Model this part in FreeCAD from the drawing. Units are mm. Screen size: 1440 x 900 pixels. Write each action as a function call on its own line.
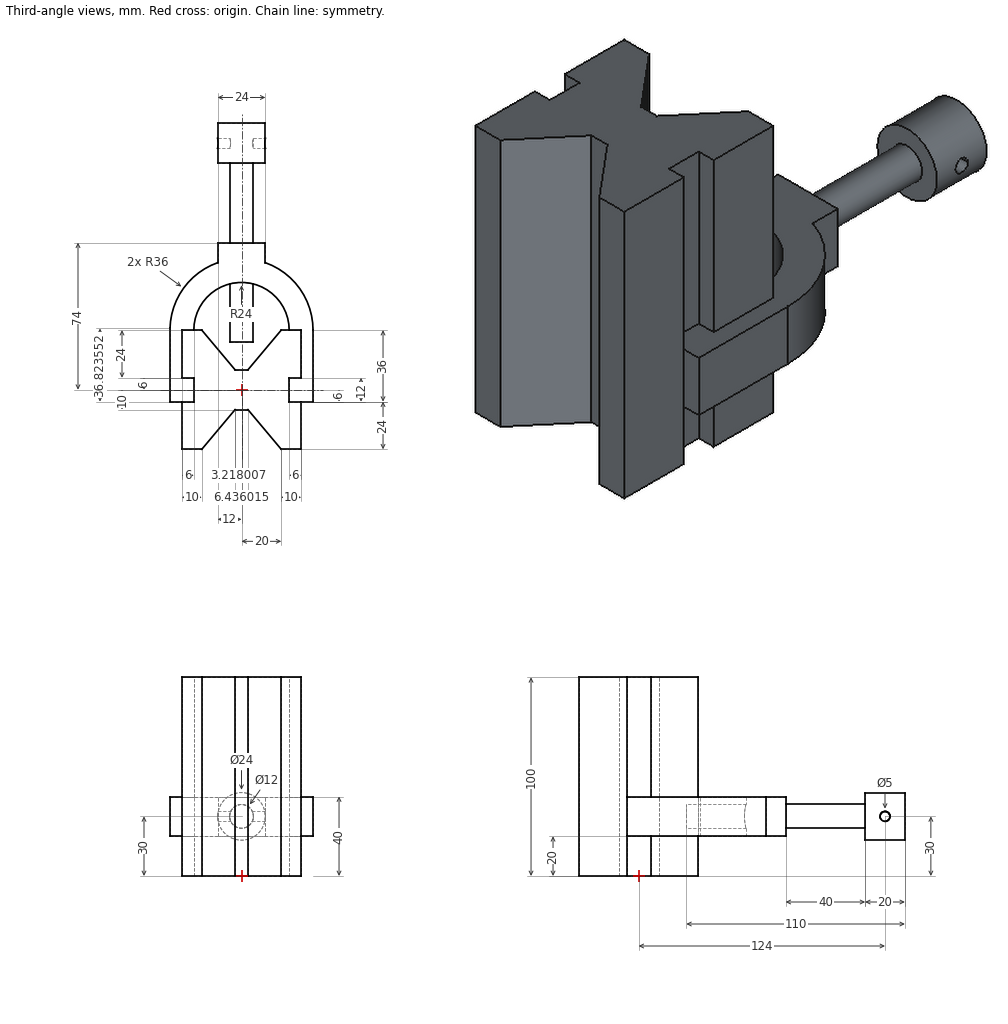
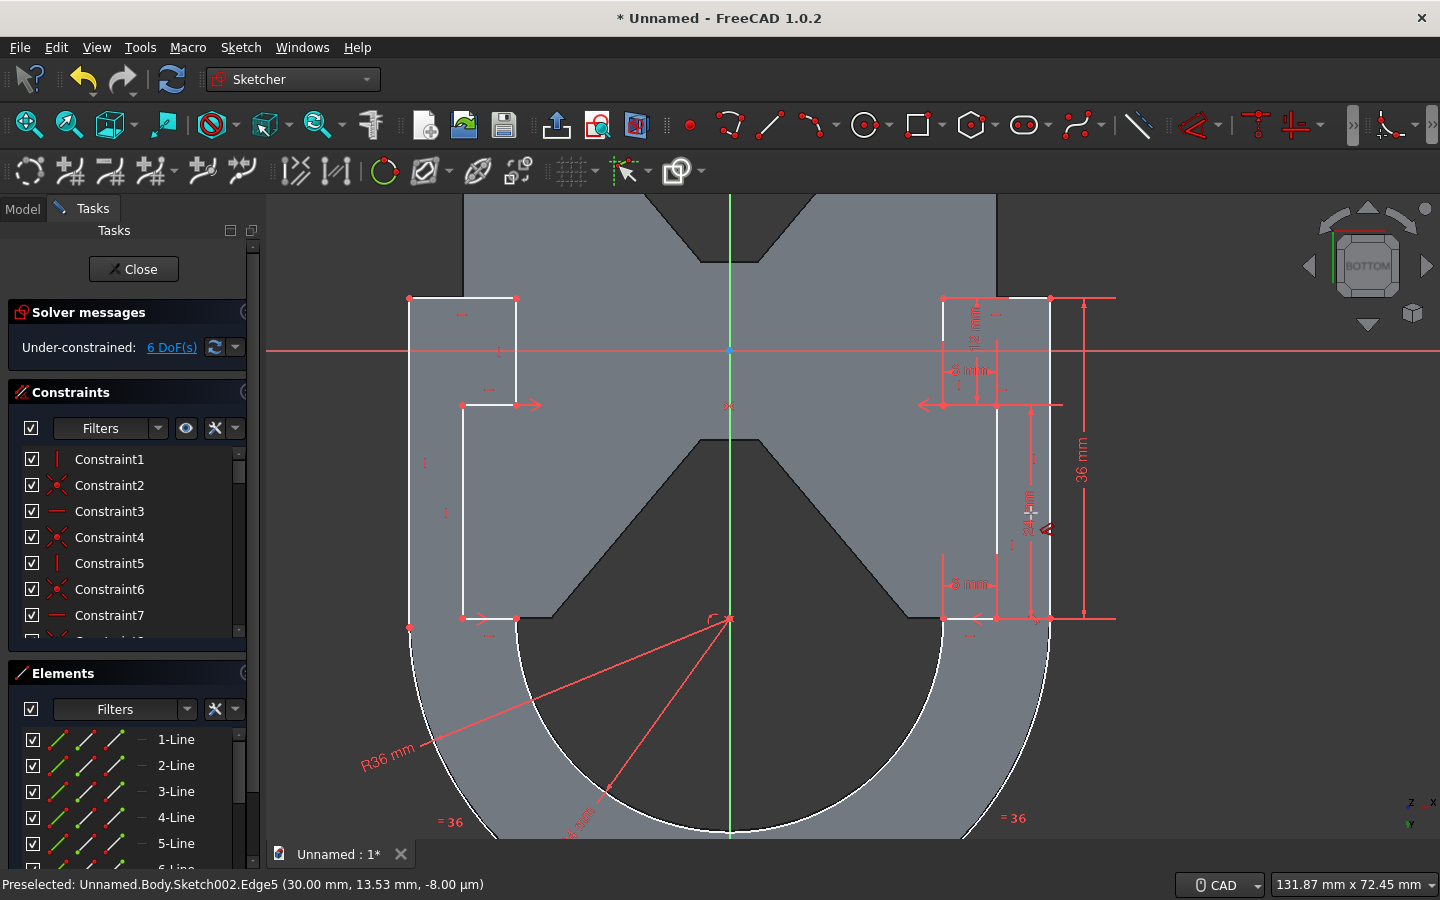
click(516, 373)
click(482, 327)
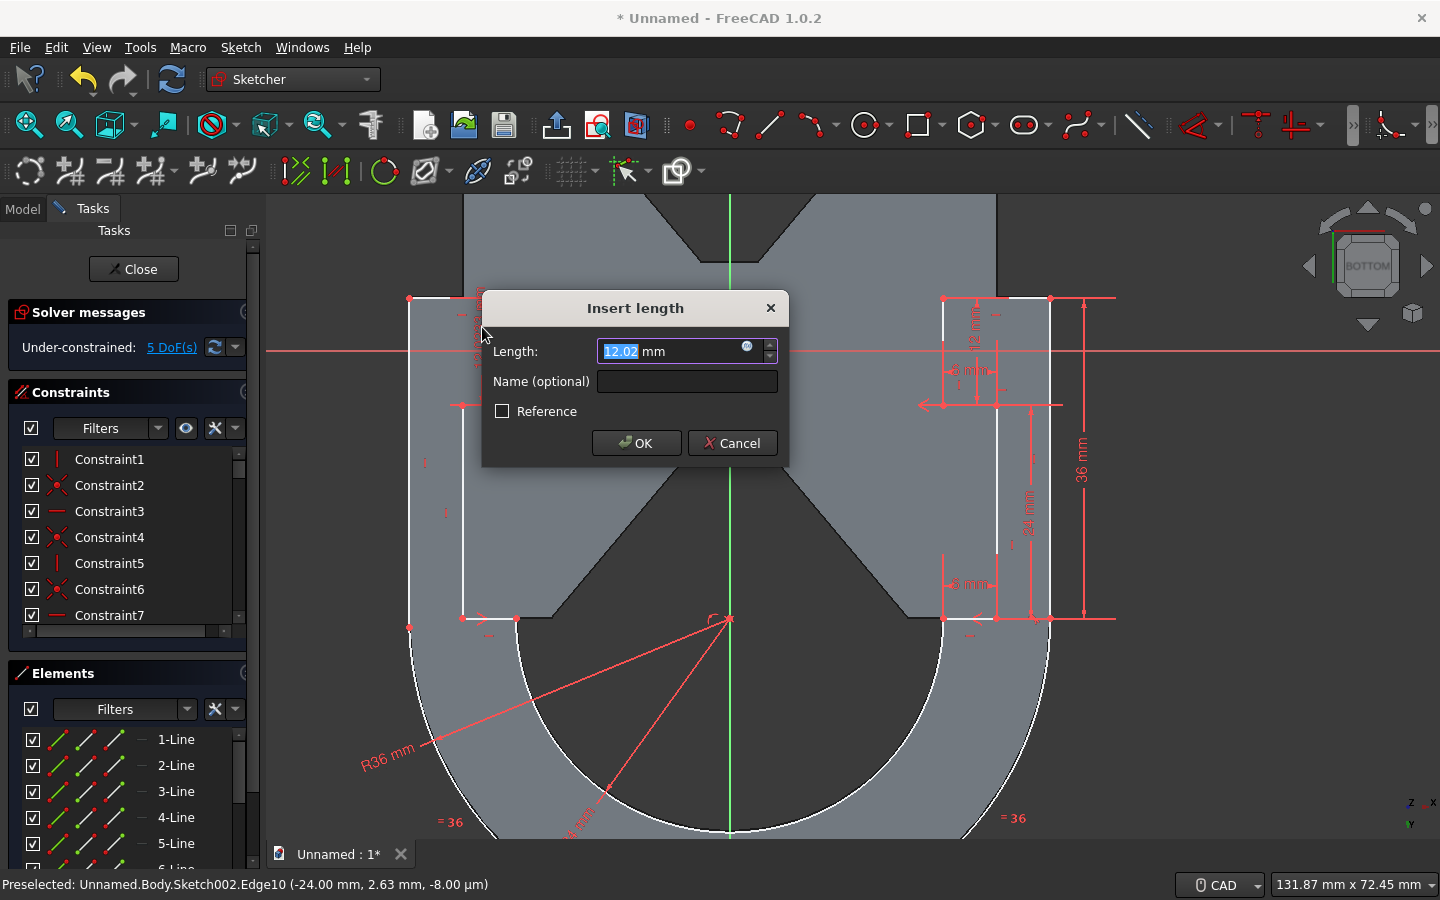
text(12)
key(Return)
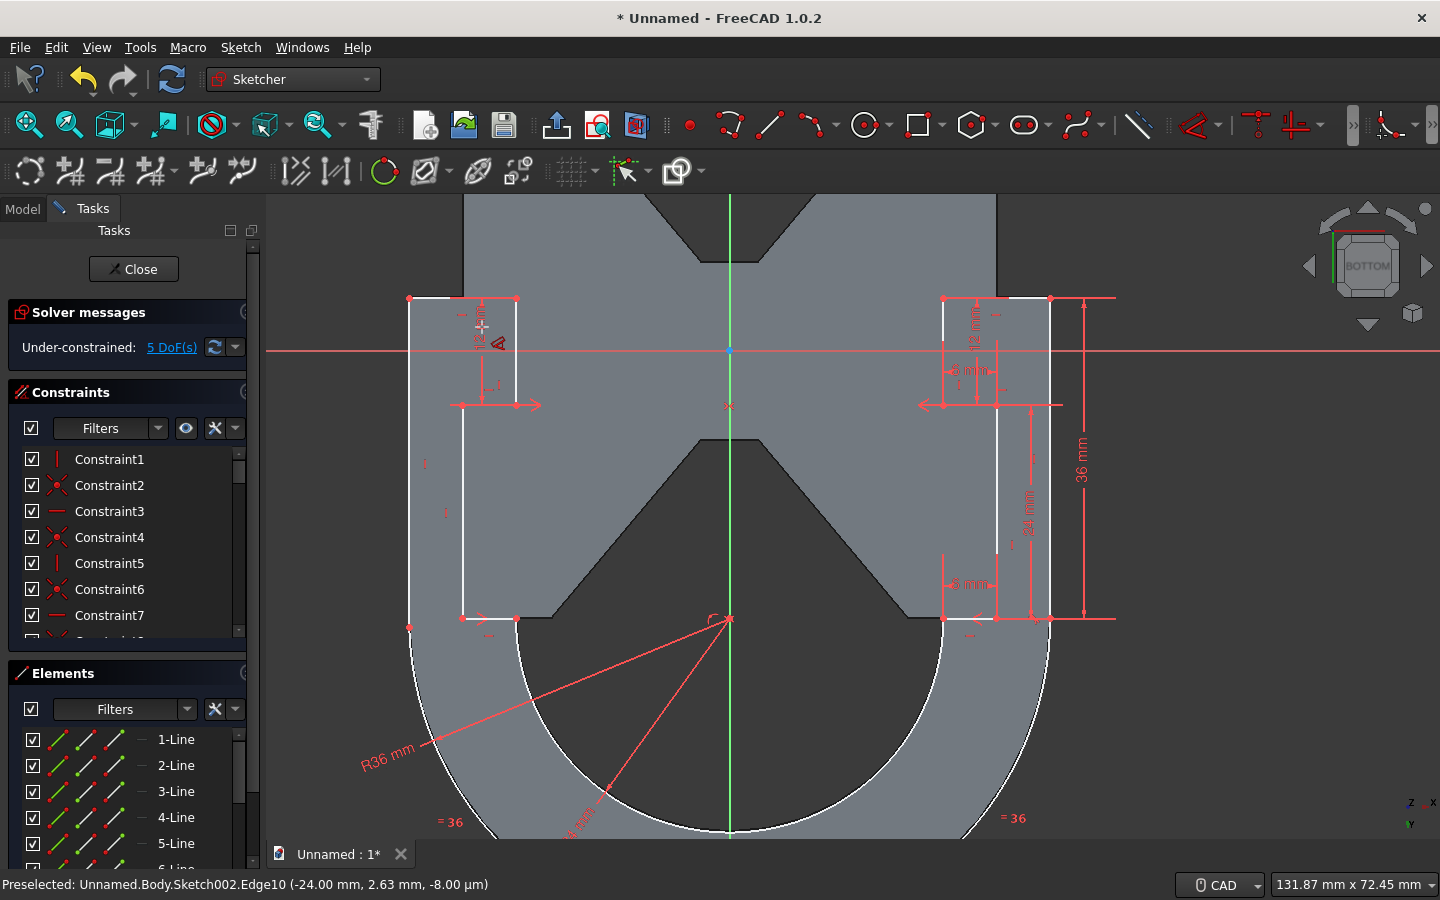
scroll(851, 350, down, 3)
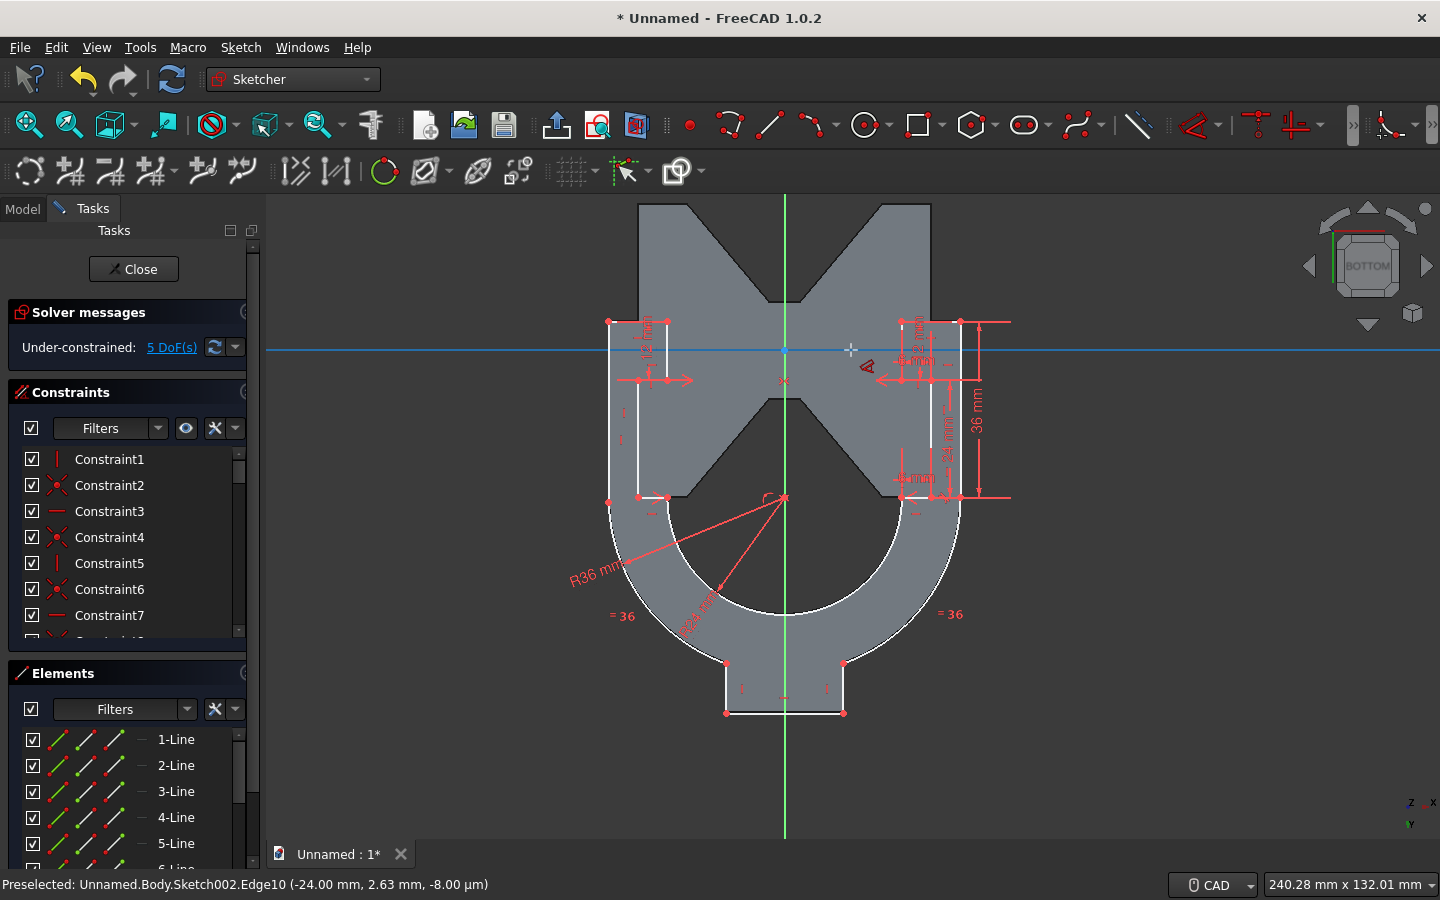
click(761, 714)
click(758, 748)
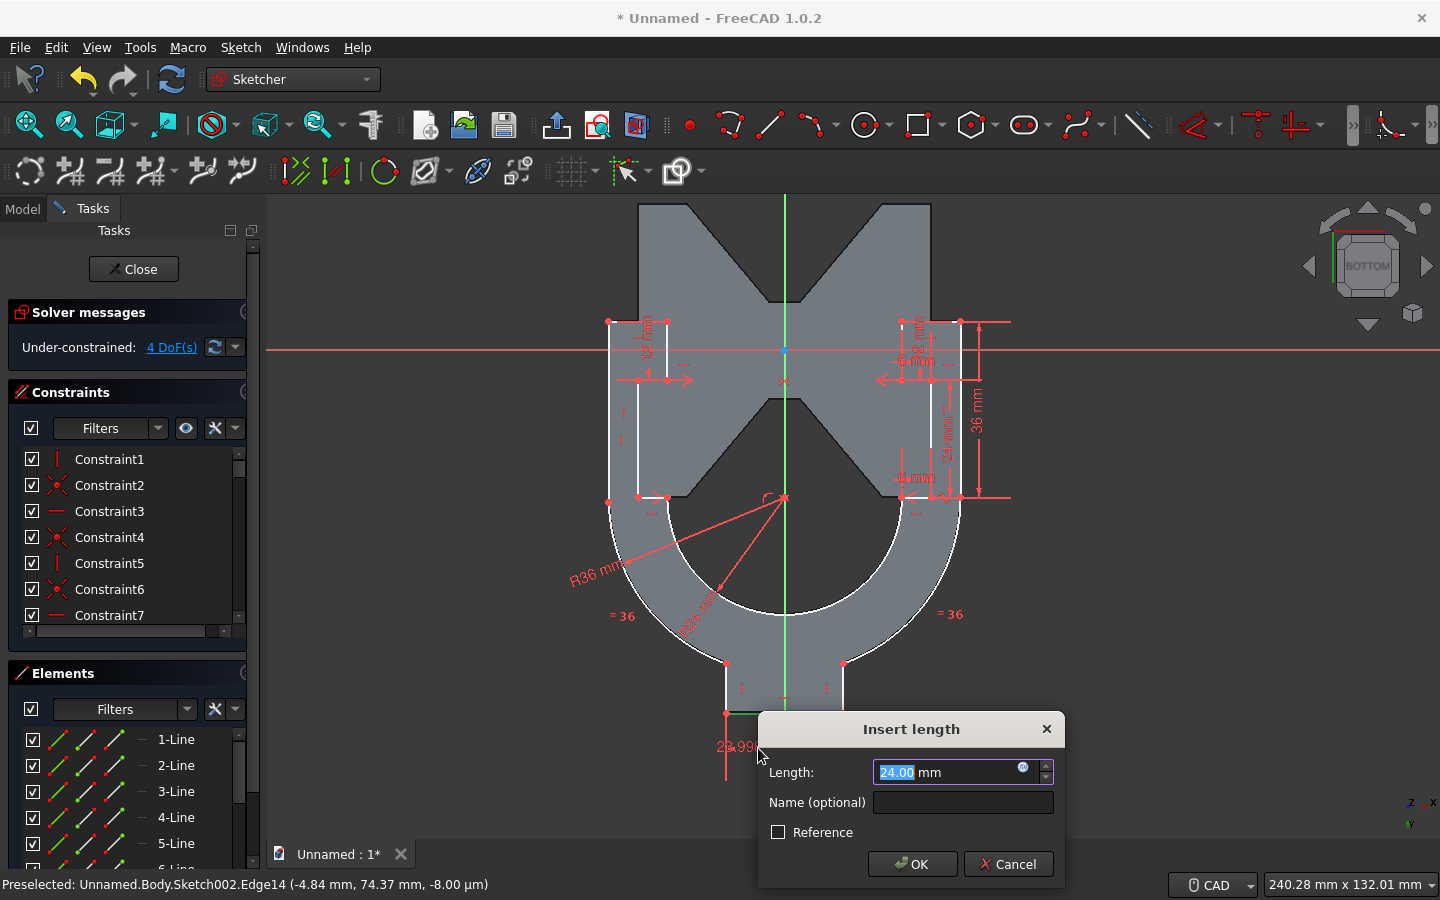
text(24)
key(Return)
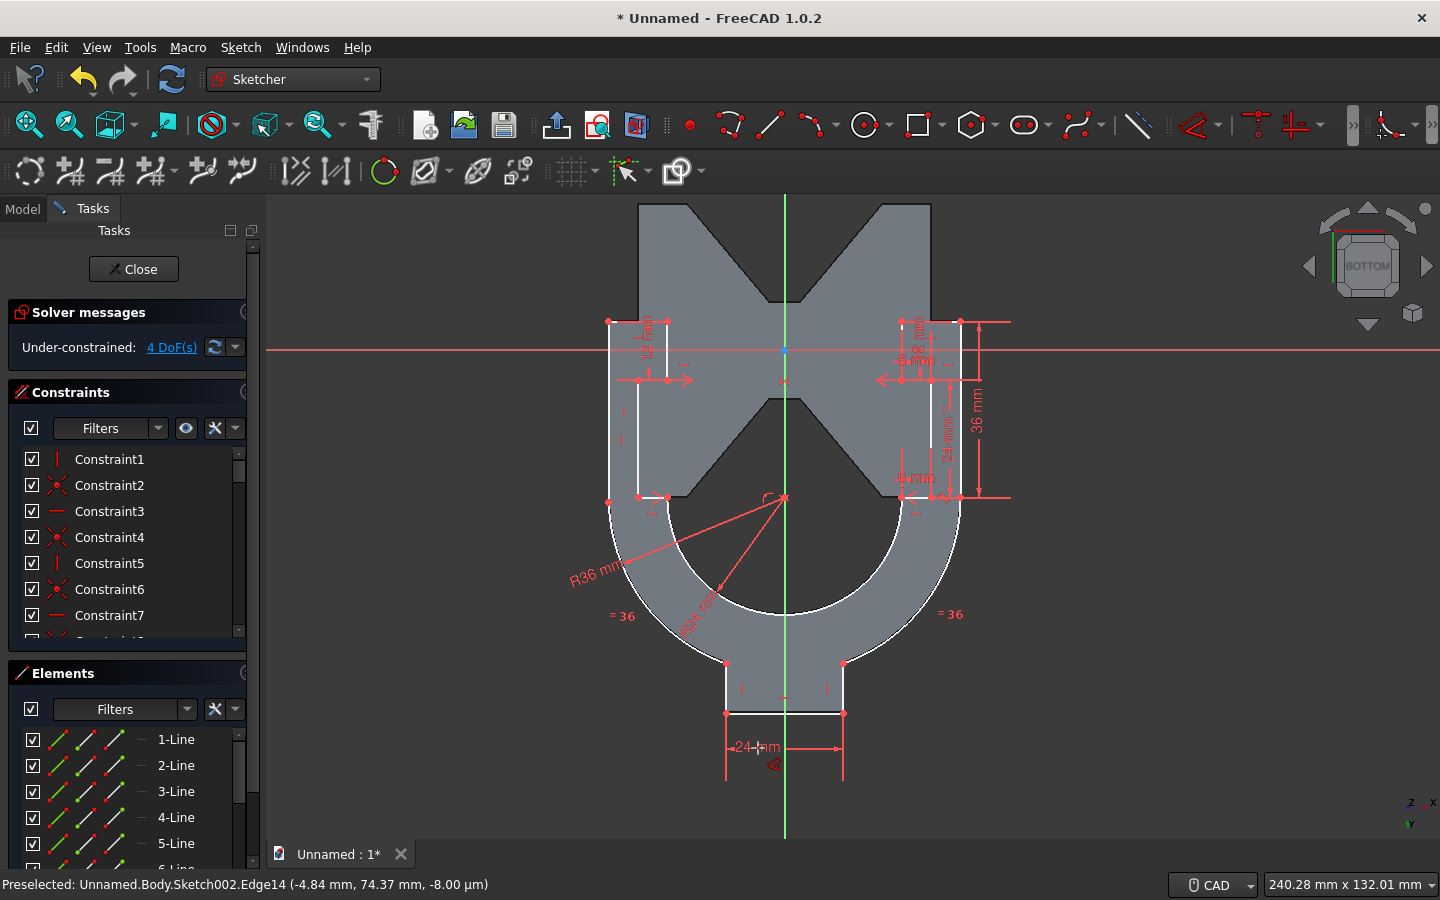
scroll(961, 322, up, 2)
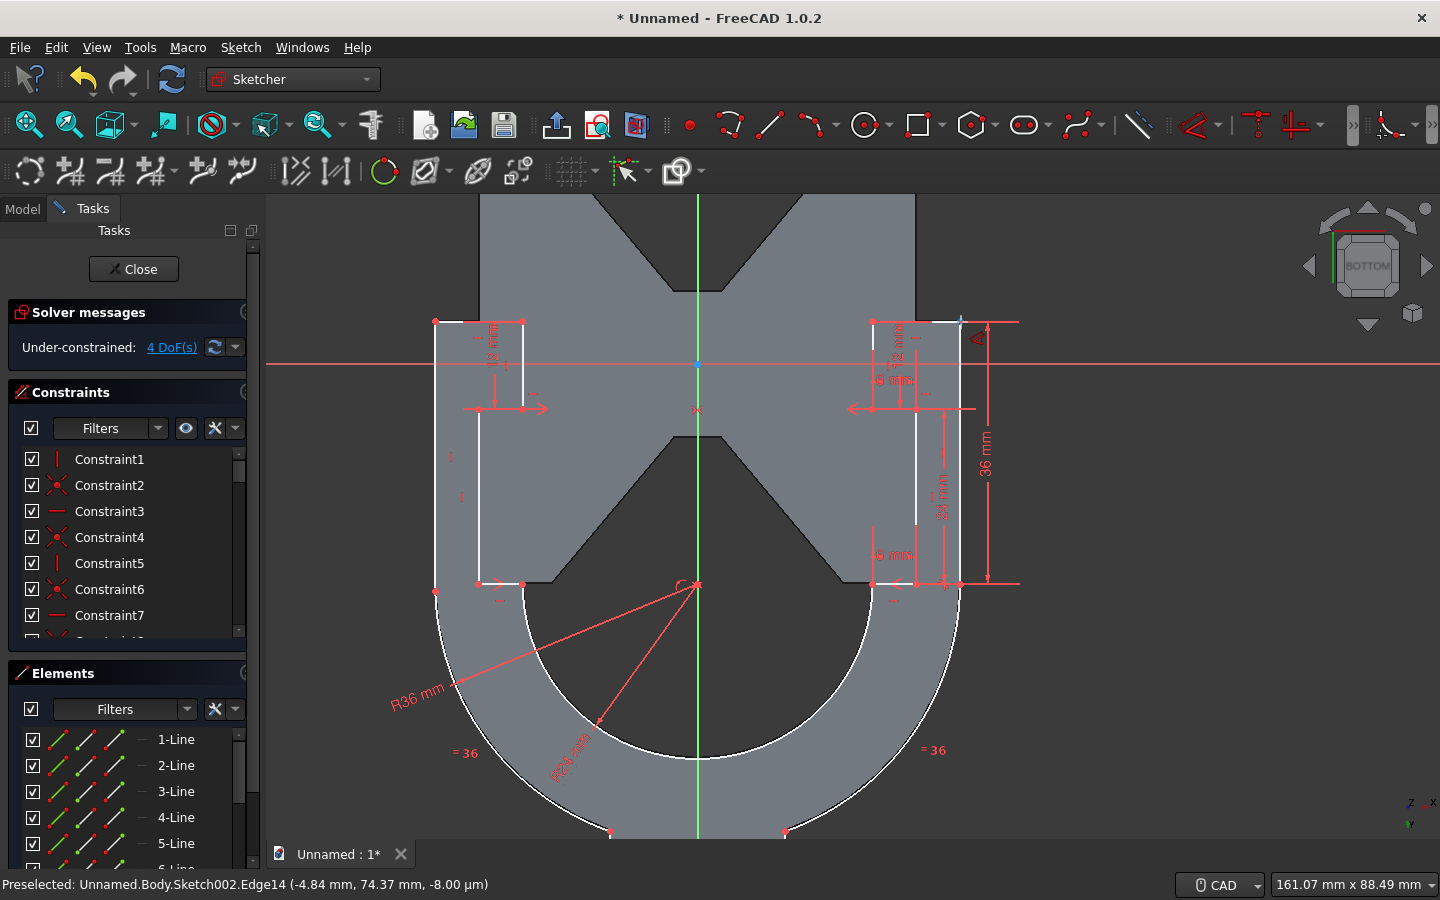
click(960, 322)
click(994, 343)